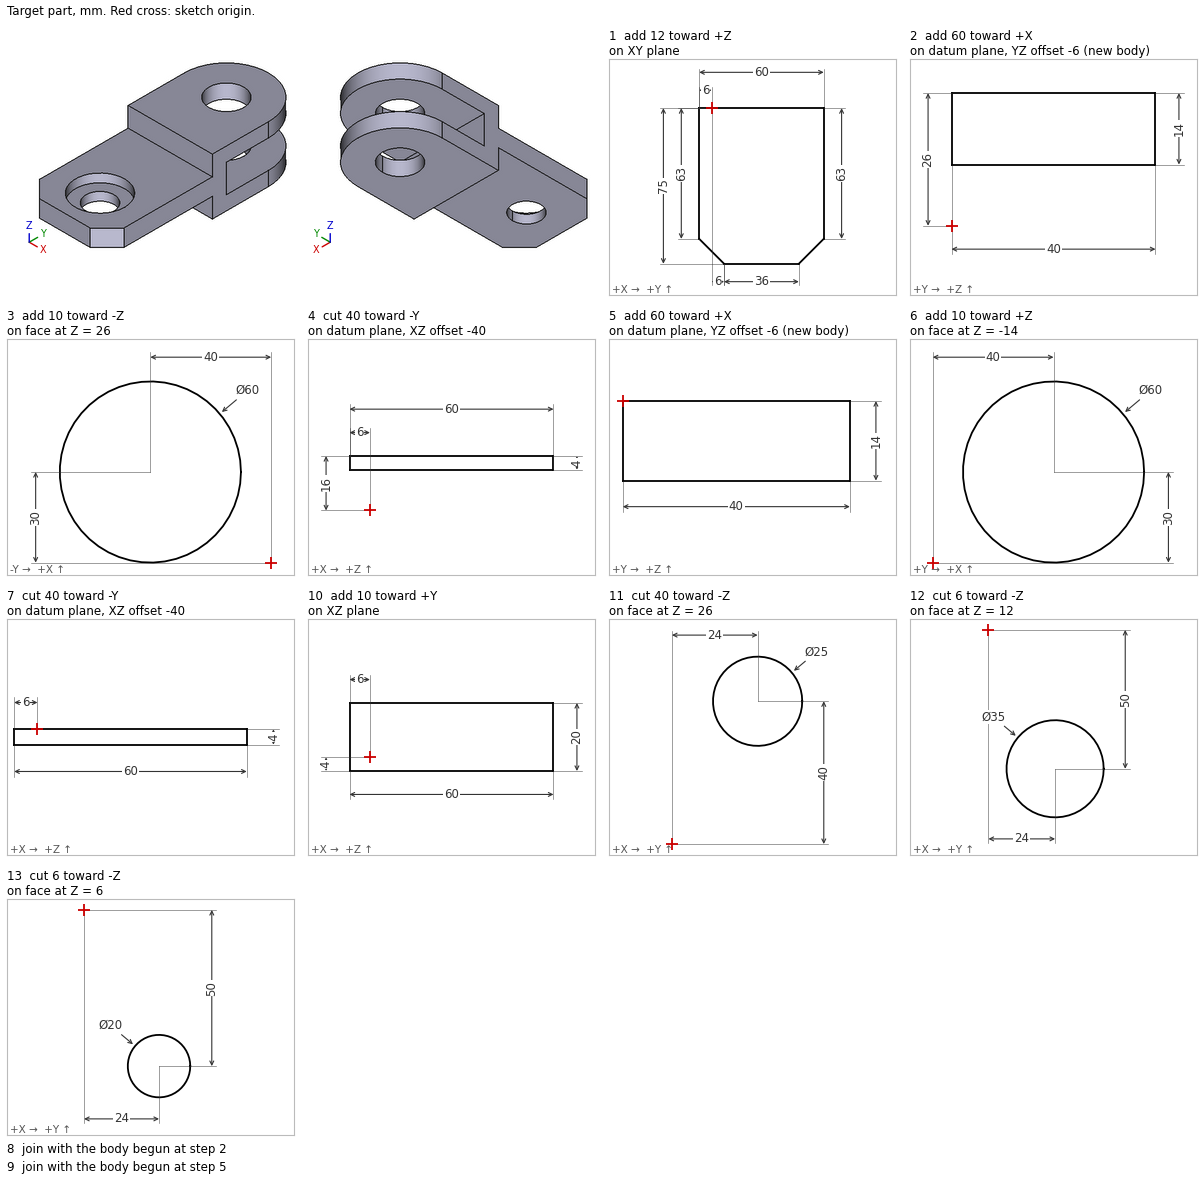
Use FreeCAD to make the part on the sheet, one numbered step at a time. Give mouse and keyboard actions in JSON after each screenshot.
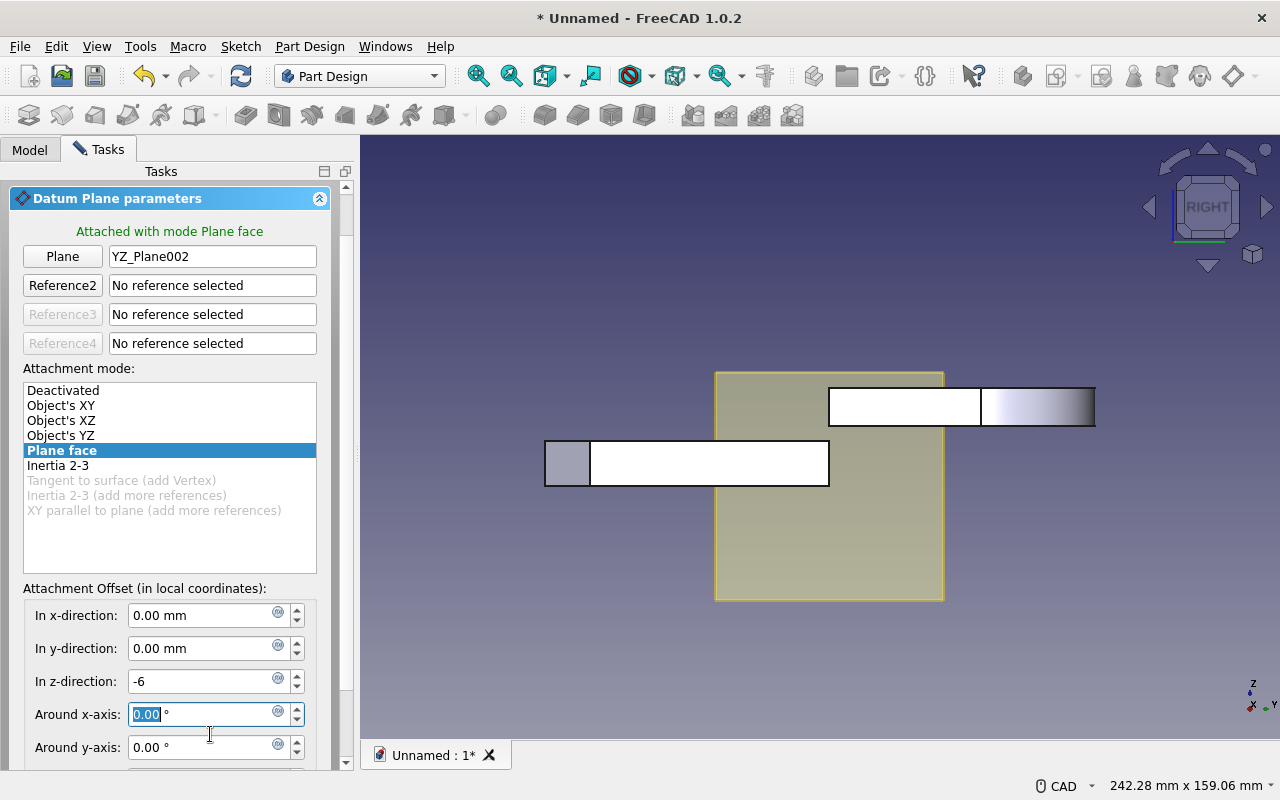
{"action": "scroll", "coordinate": [346, 476], "scroll_direction": "up", "scroll_amount": 2}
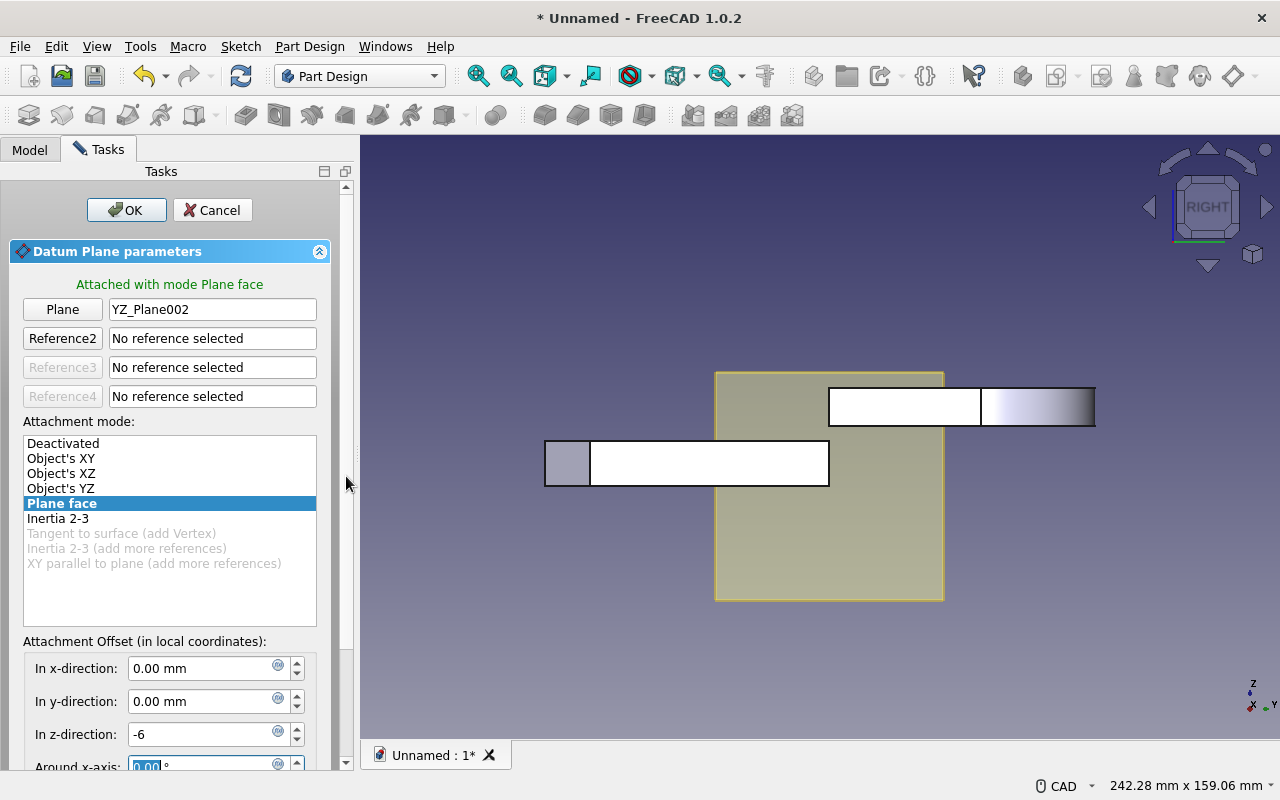
{"action": "left_click", "coordinate": [127, 210]}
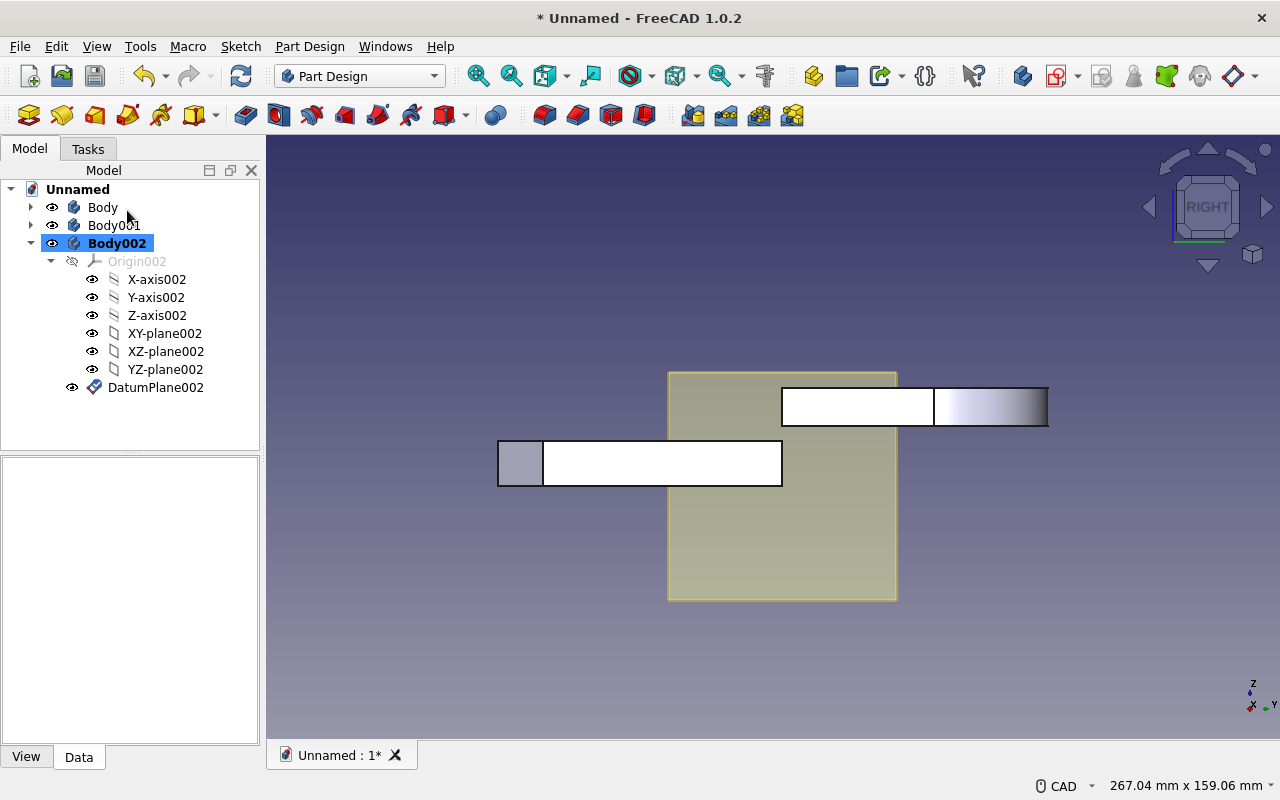
{"action": "left_click", "coordinate": [117, 387]}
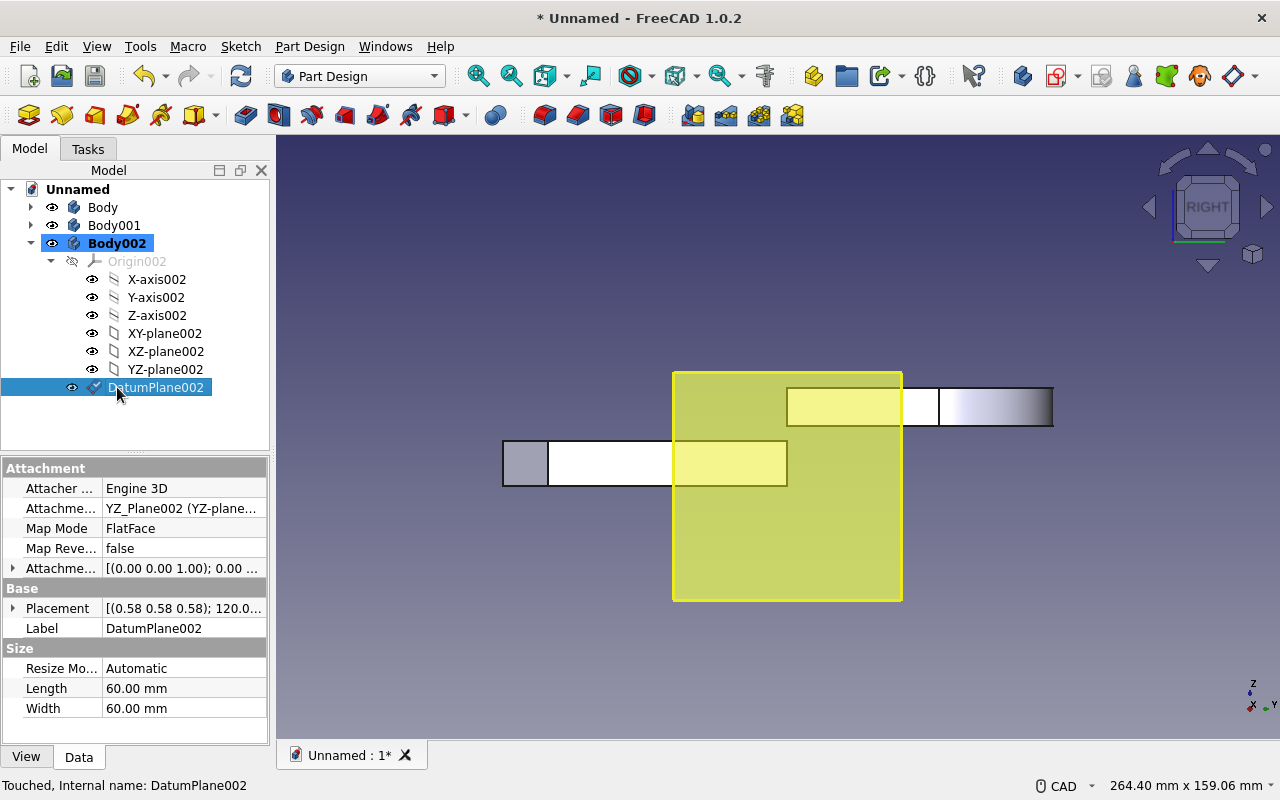
{"action": "left_click", "coordinate": [1056, 76]}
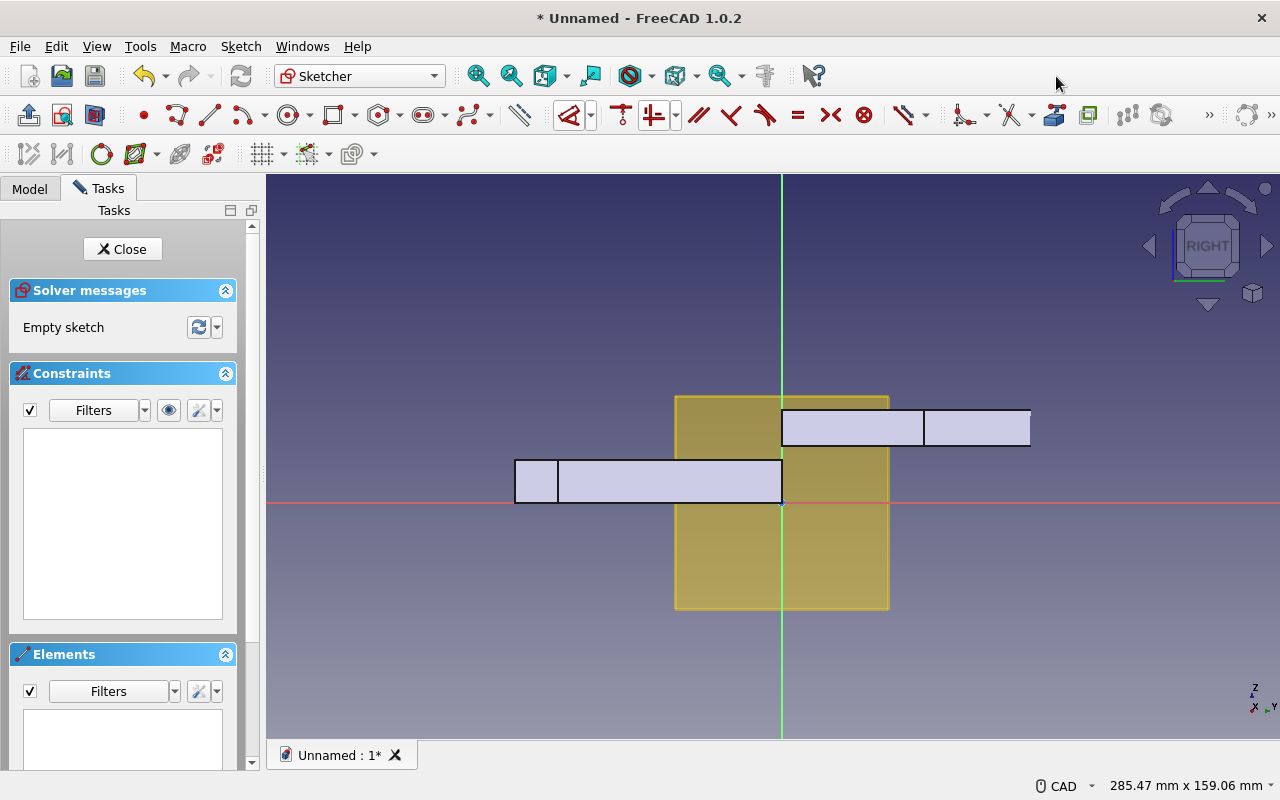
{"action": "scroll", "coordinate": [902, 551], "scroll_direction": "up", "scroll_amount": 7}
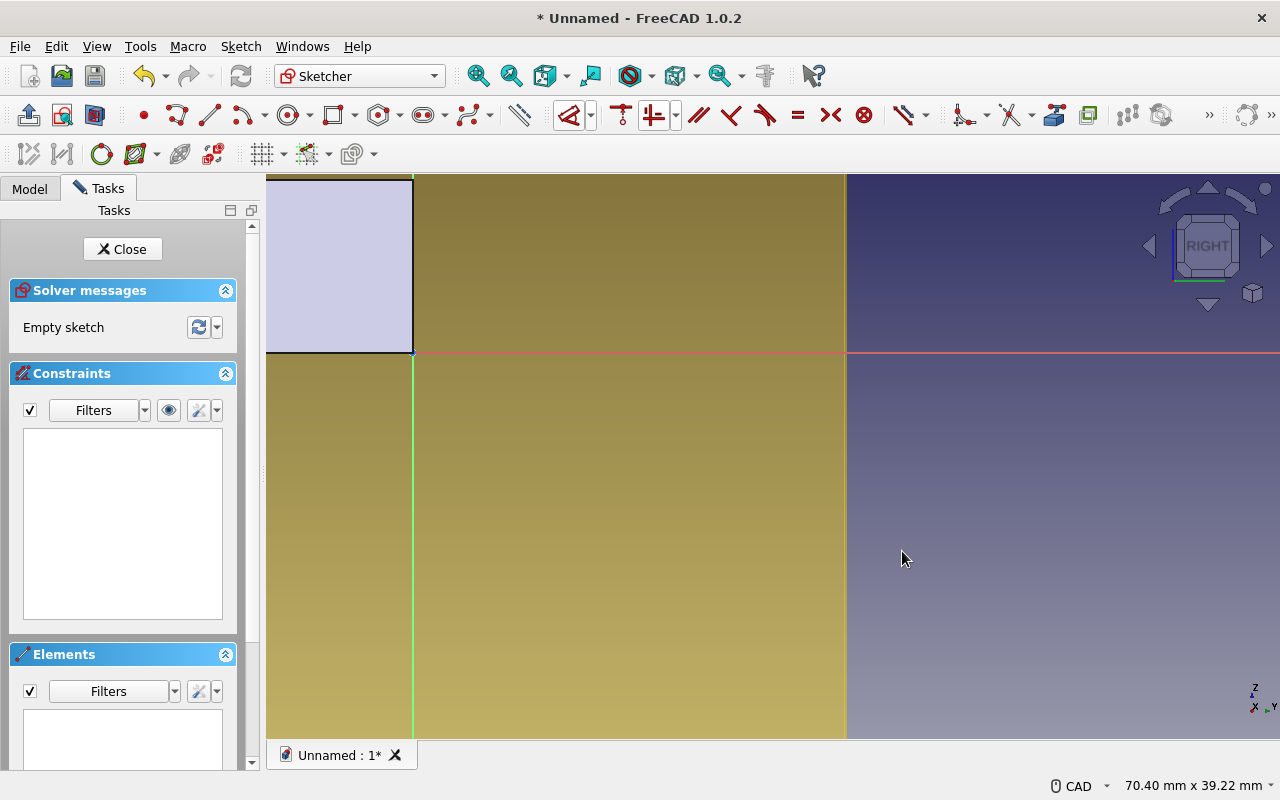
{"action": "left_click", "coordinate": [332, 116]}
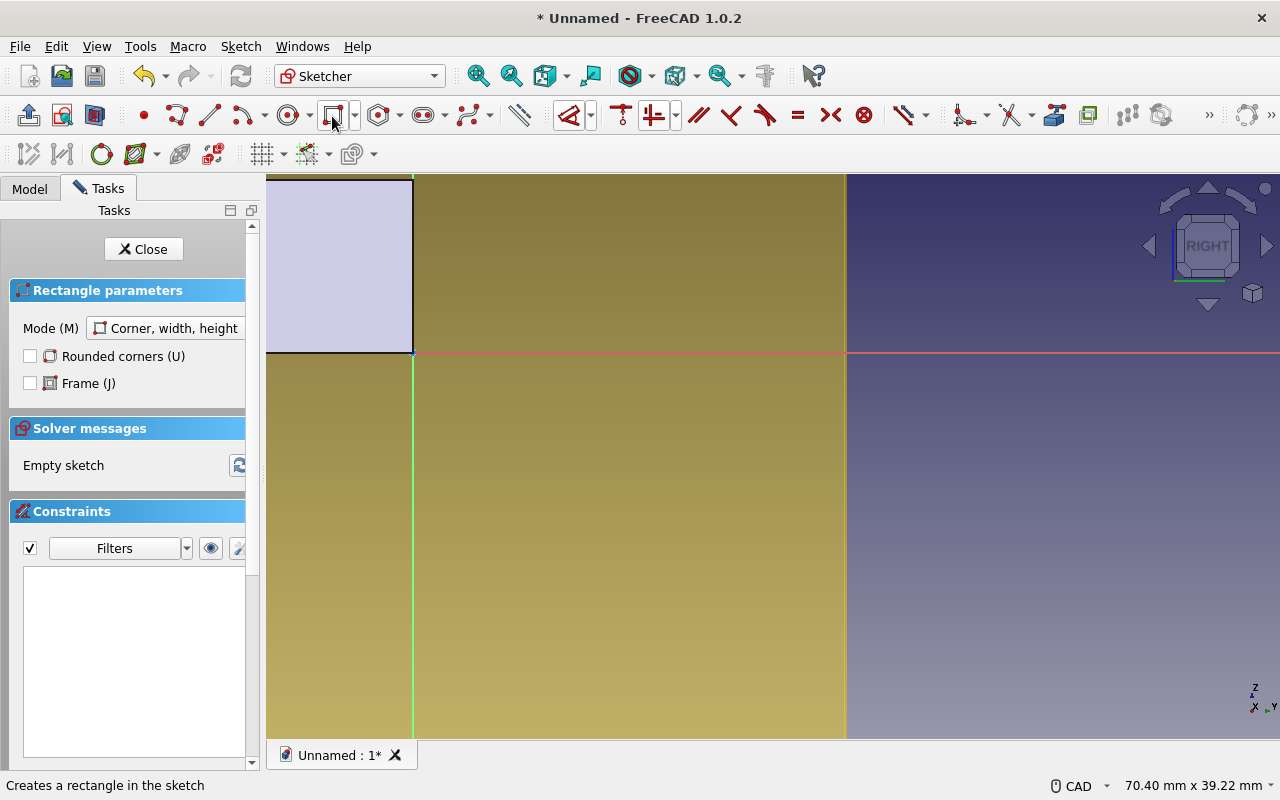
{"action": "left_click", "coordinate": [413, 353]}
{"action": "mouse_move", "coordinate": [989, 555]}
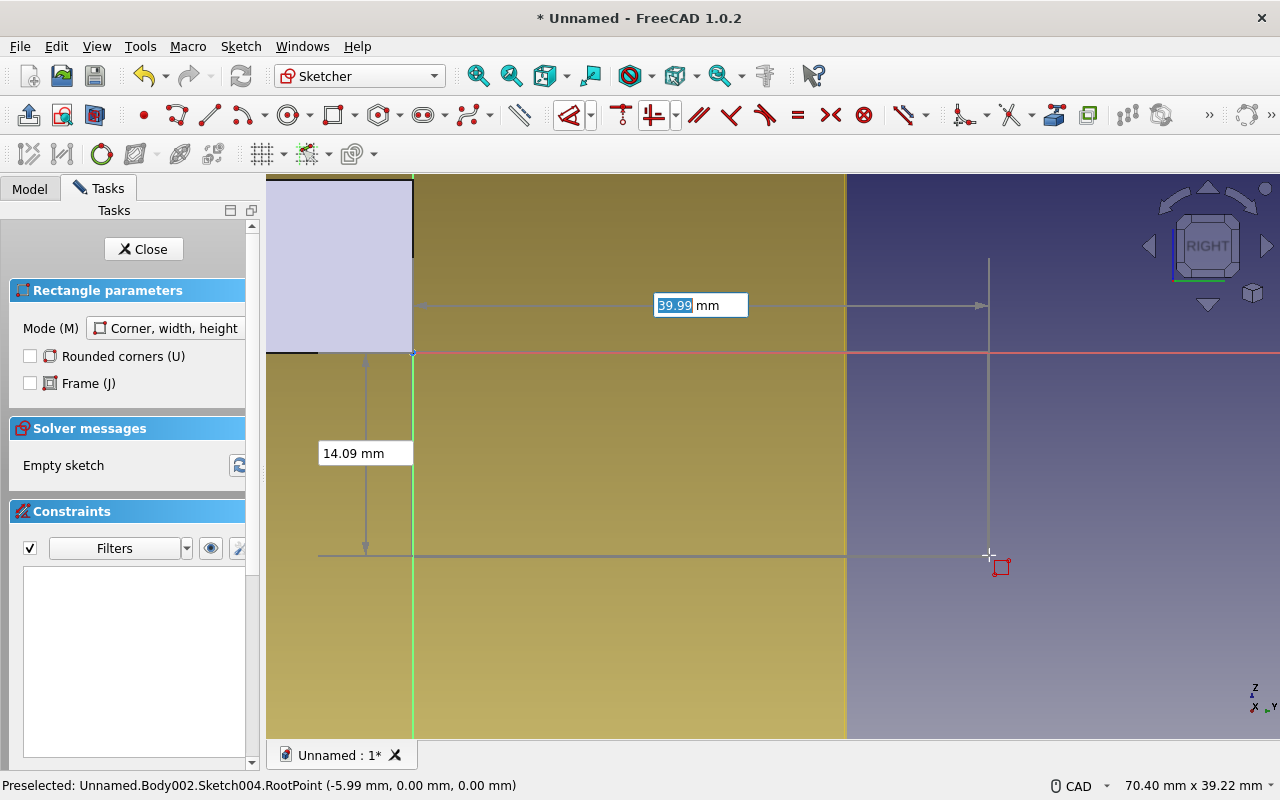
{"action": "type", "text": "40"}
{"action": "key", "text": "Tab"}
{"action": "type", "text": "14"}
{"action": "key", "text": "Return"}
{"action": "key", "text": "Escape"}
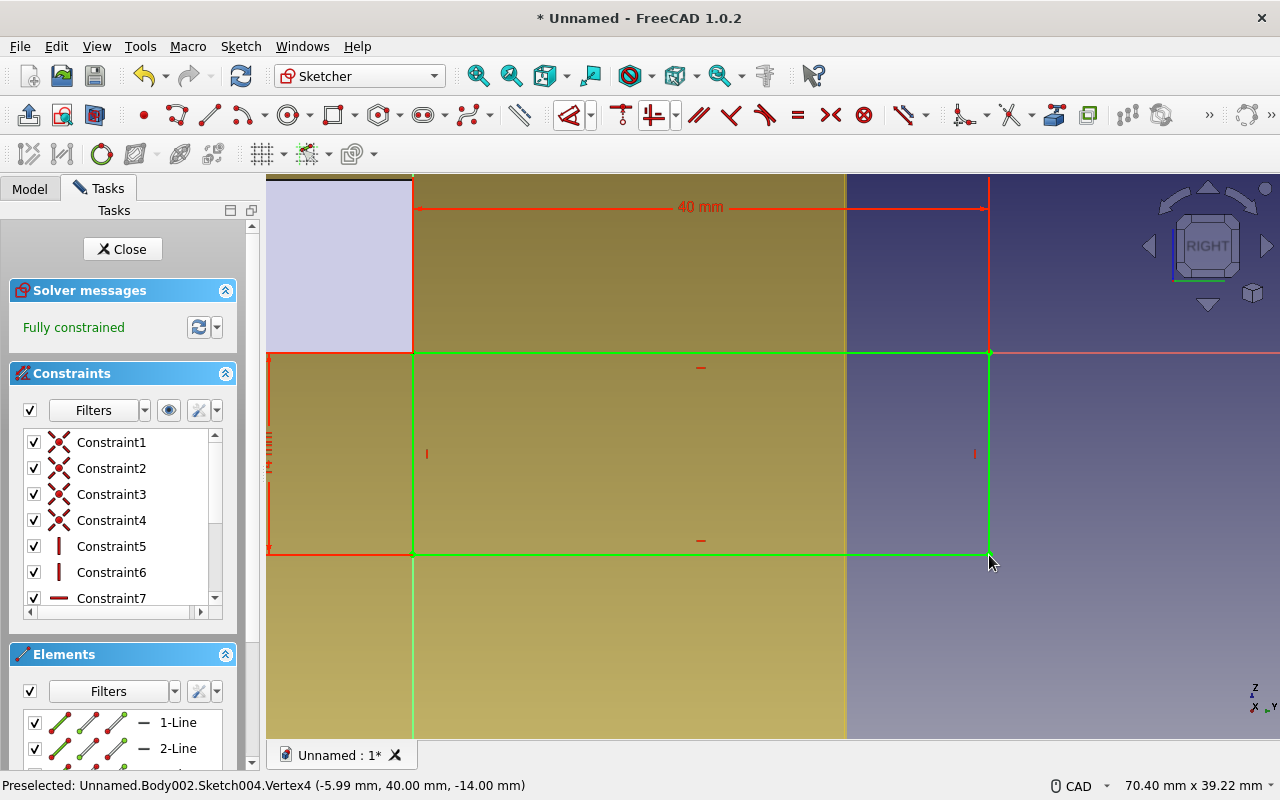
{"action": "left_click", "coordinate": [123, 249]}